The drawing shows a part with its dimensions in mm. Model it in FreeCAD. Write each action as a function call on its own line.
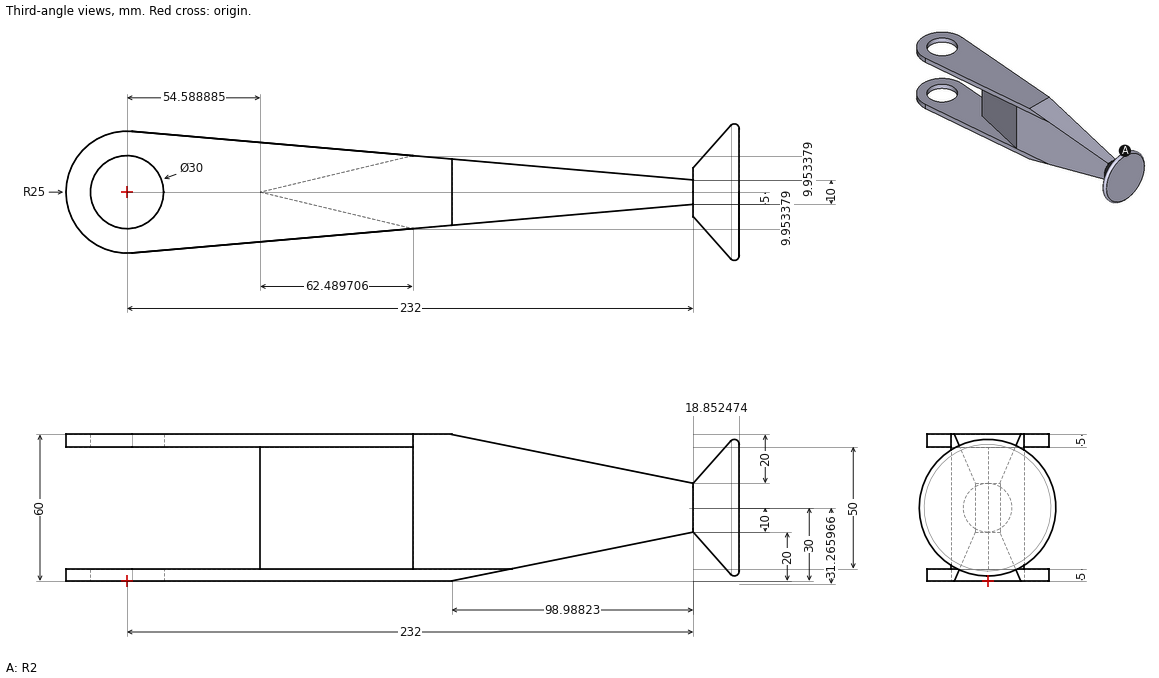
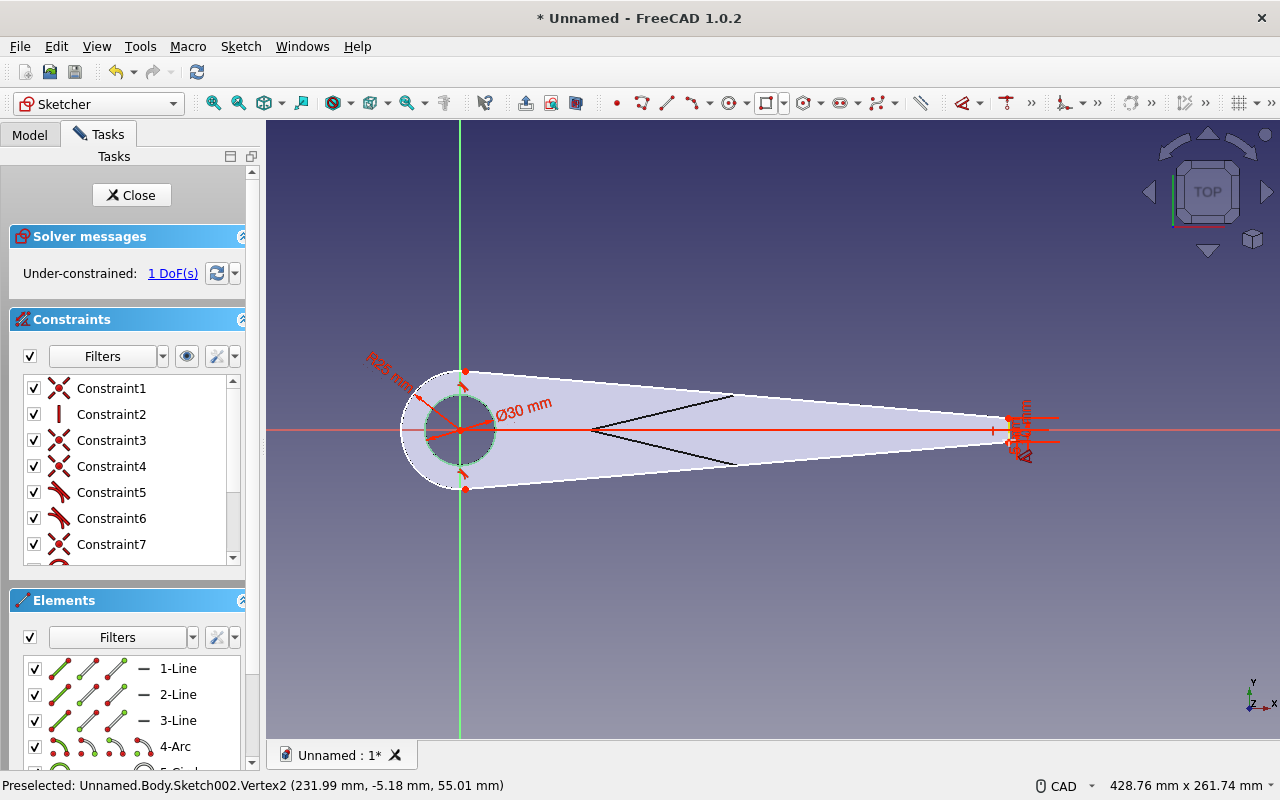
click(1009, 442)
click(861, 476)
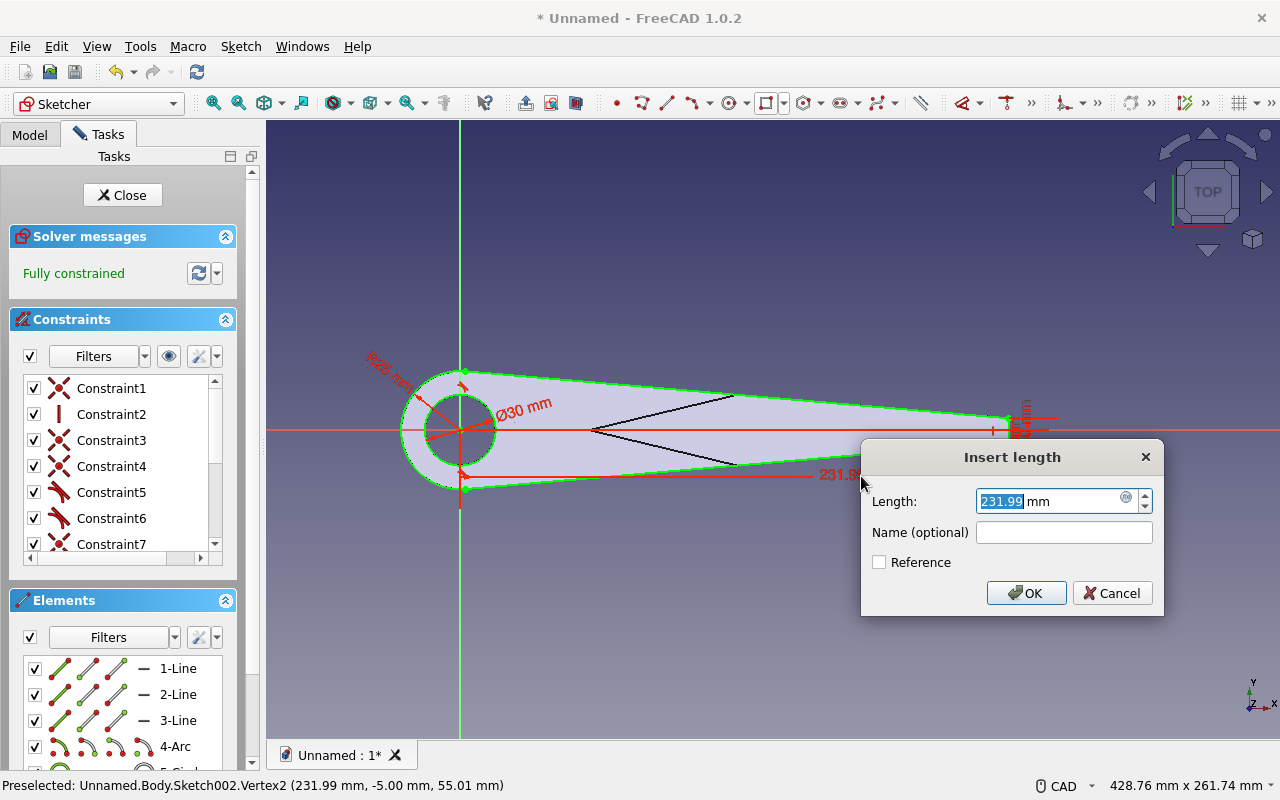
text(232)
key(Return)
key(Escape)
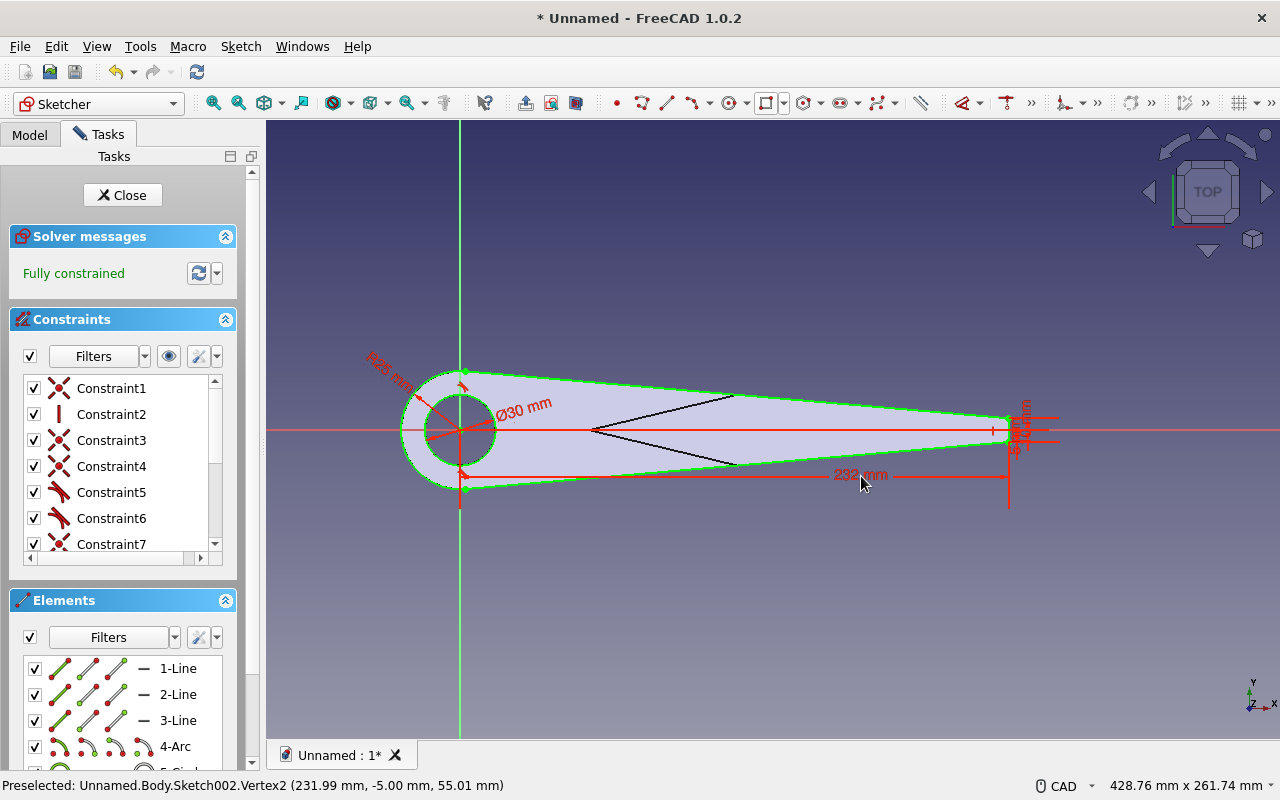
click(123, 195)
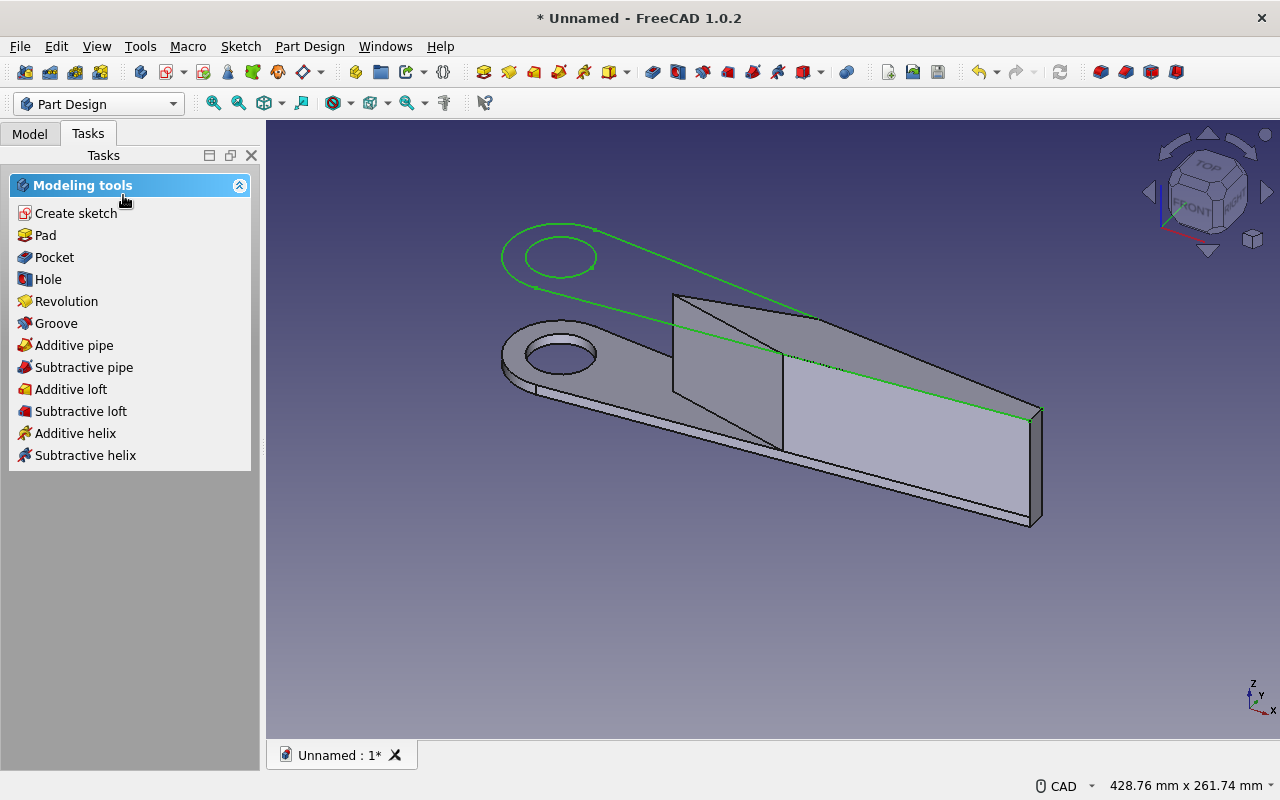
click(484, 72)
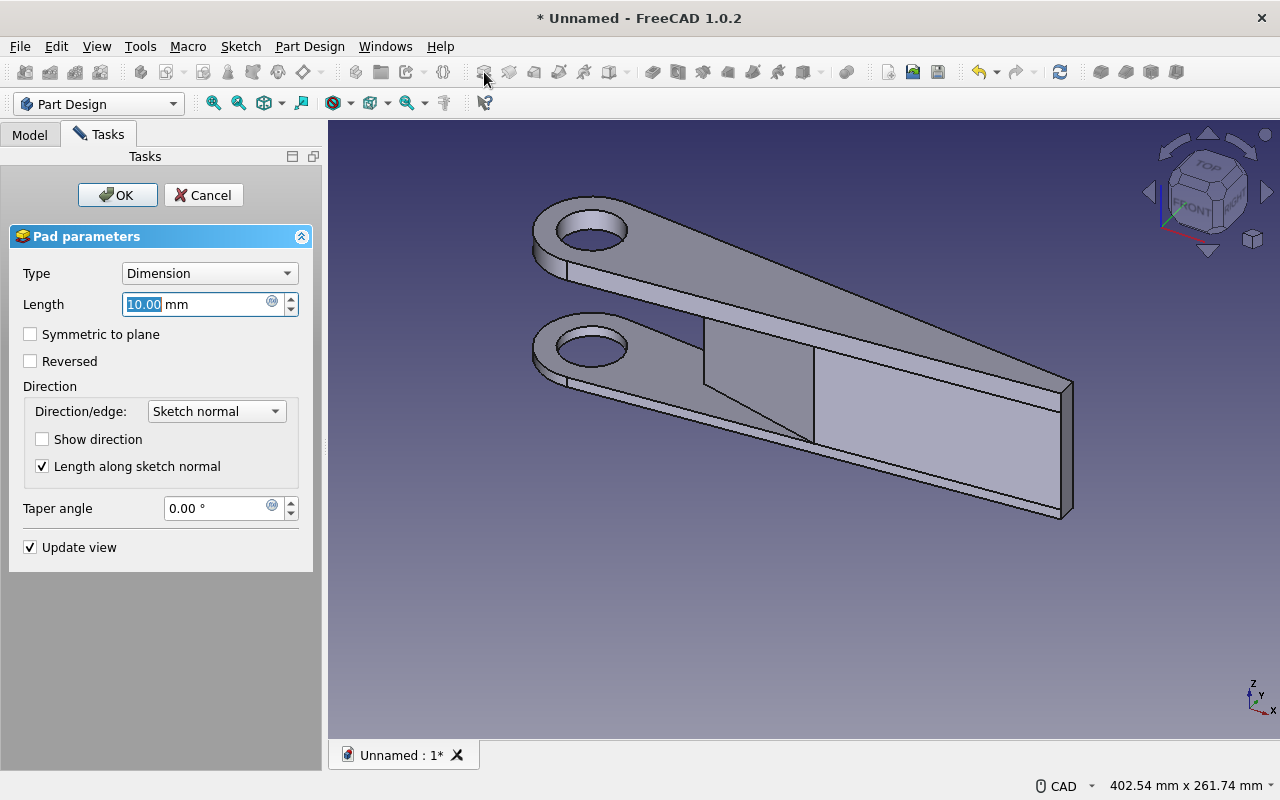
text(5)
key(Tab)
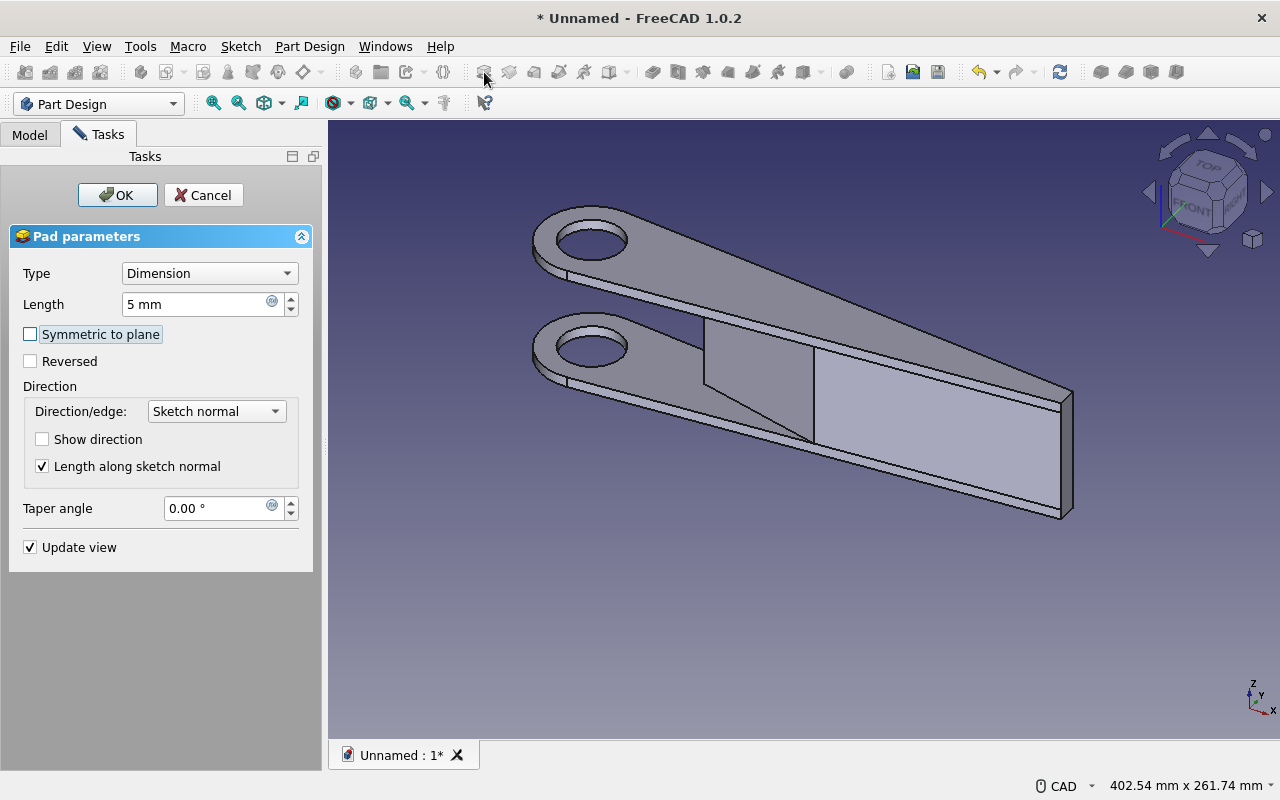
click(118, 195)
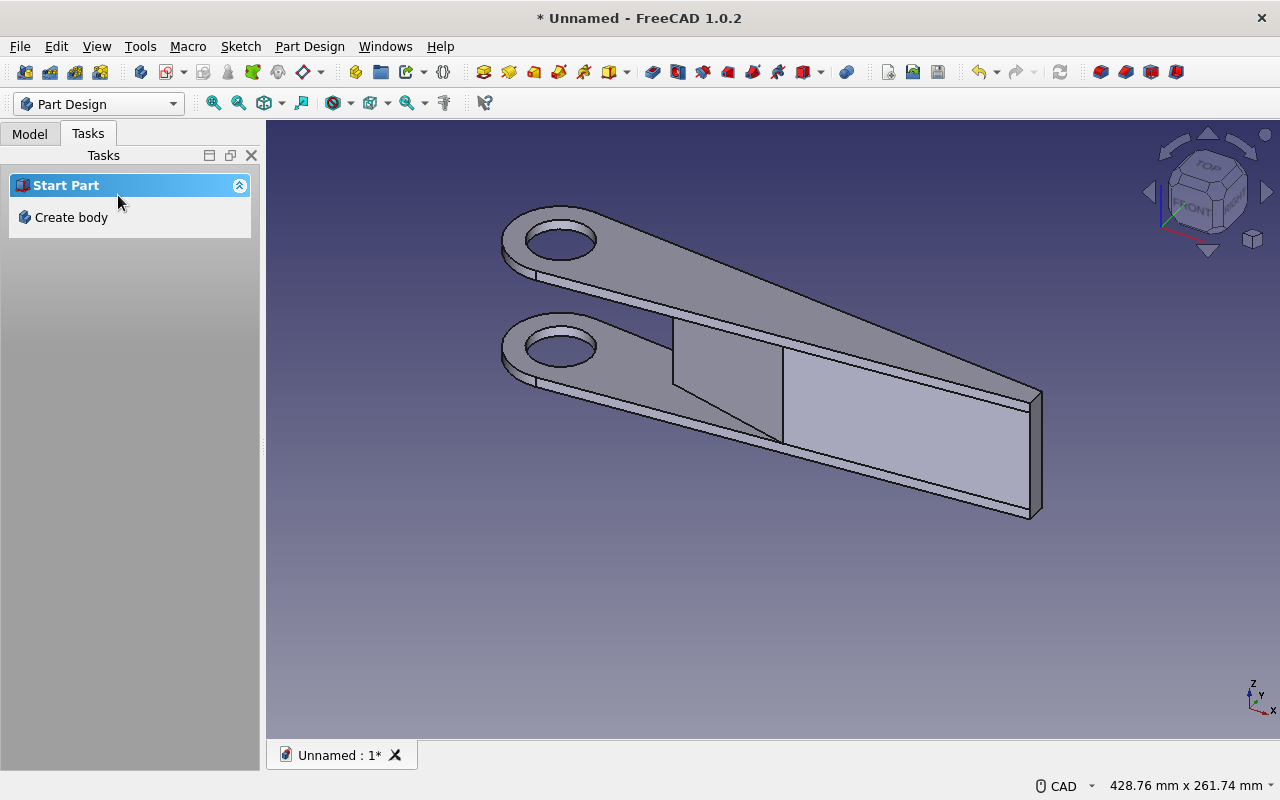
click(166, 72)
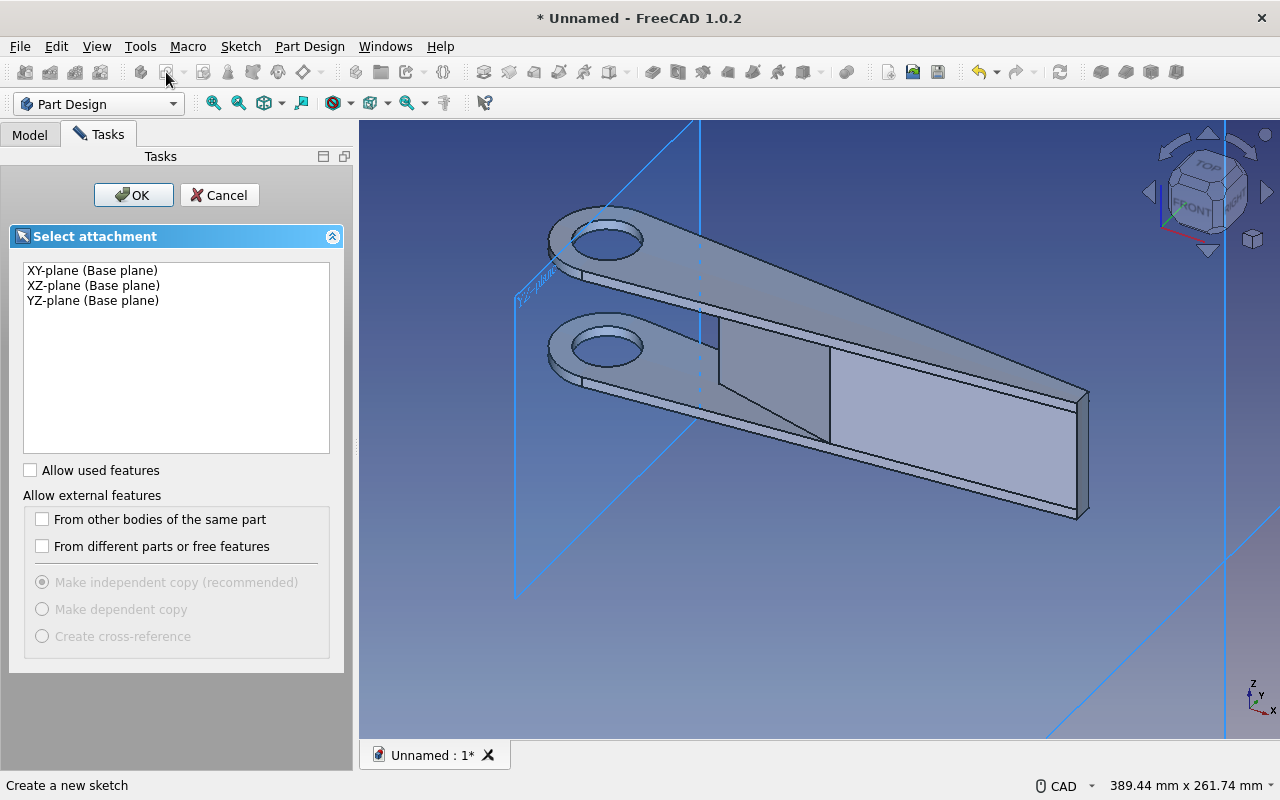
click(84, 286)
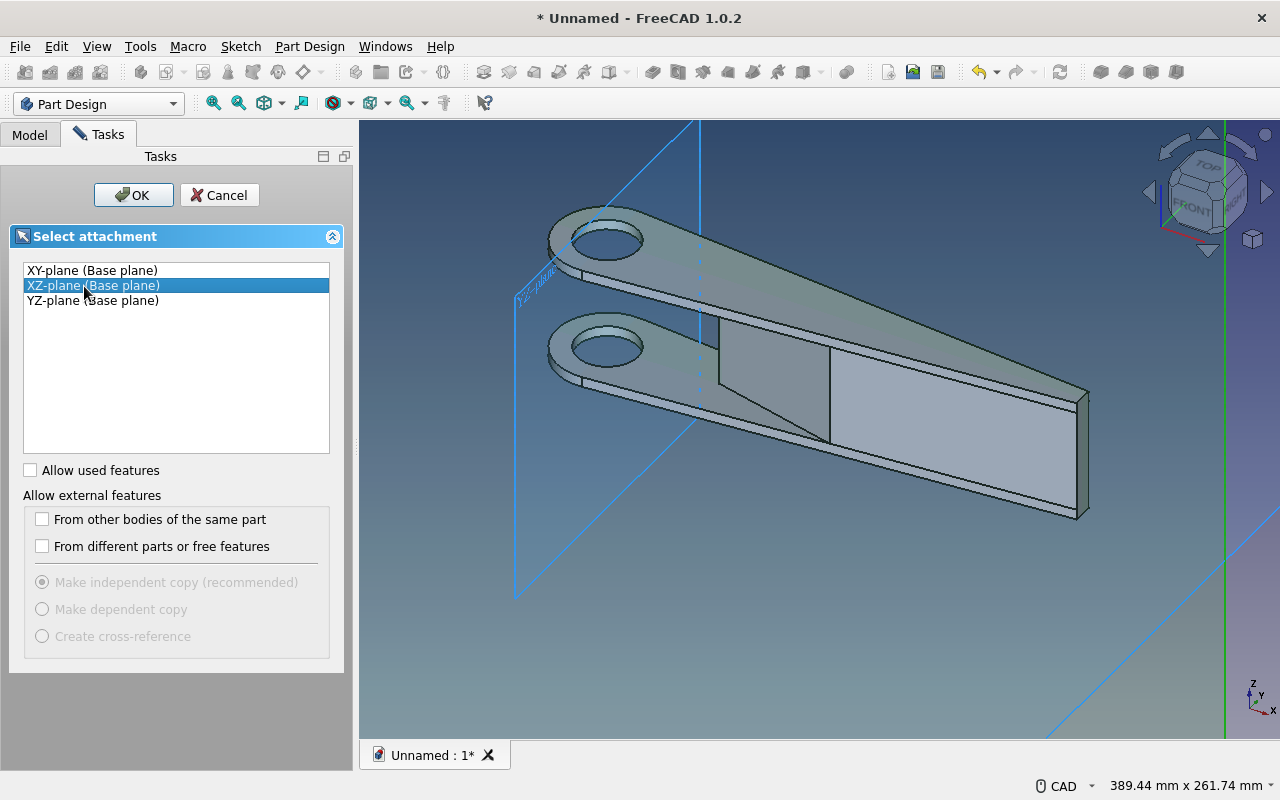
click(134, 195)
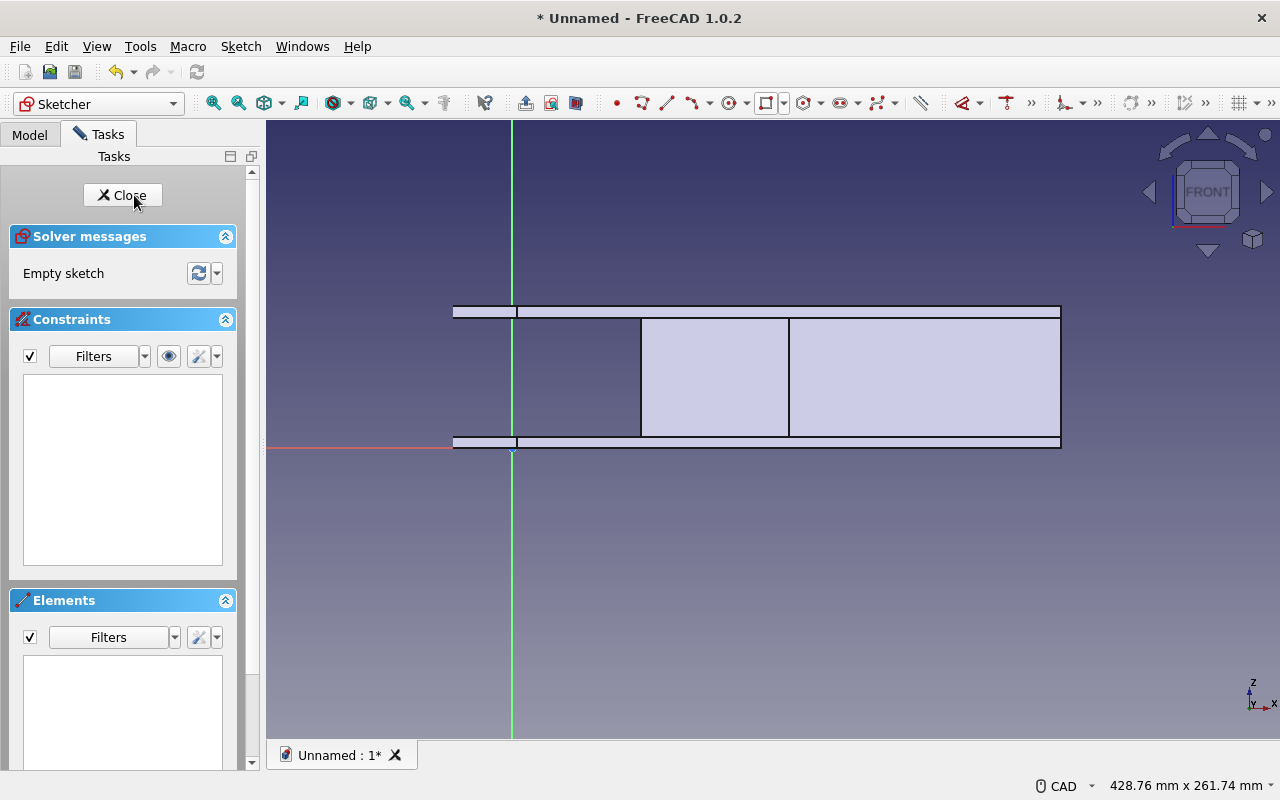
click(576, 104)